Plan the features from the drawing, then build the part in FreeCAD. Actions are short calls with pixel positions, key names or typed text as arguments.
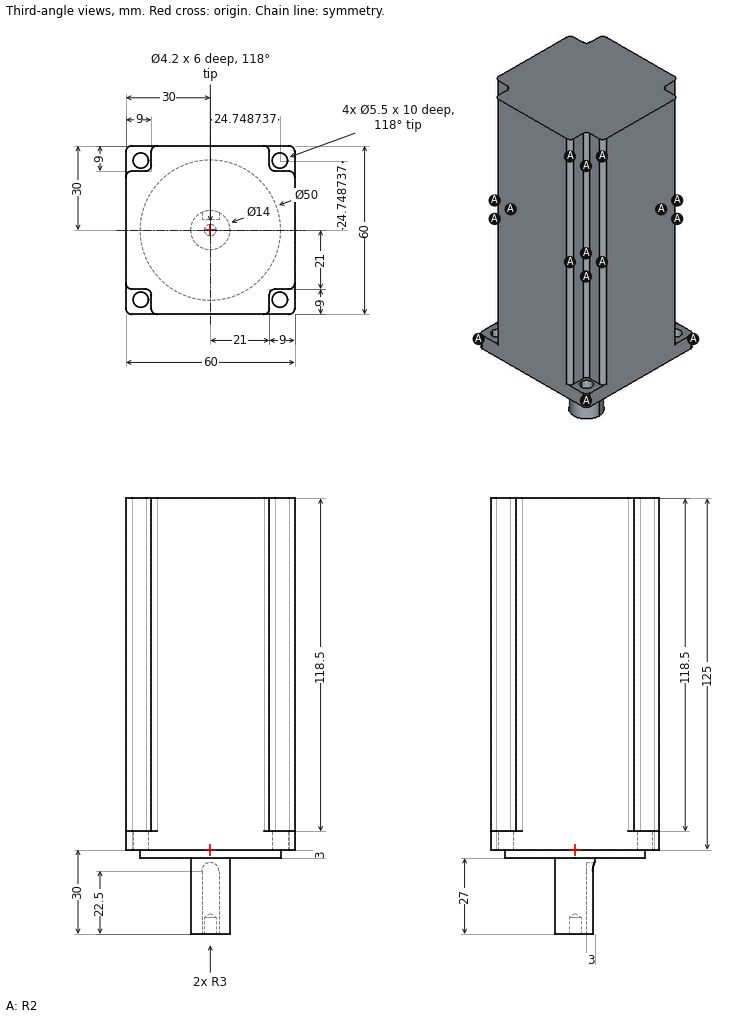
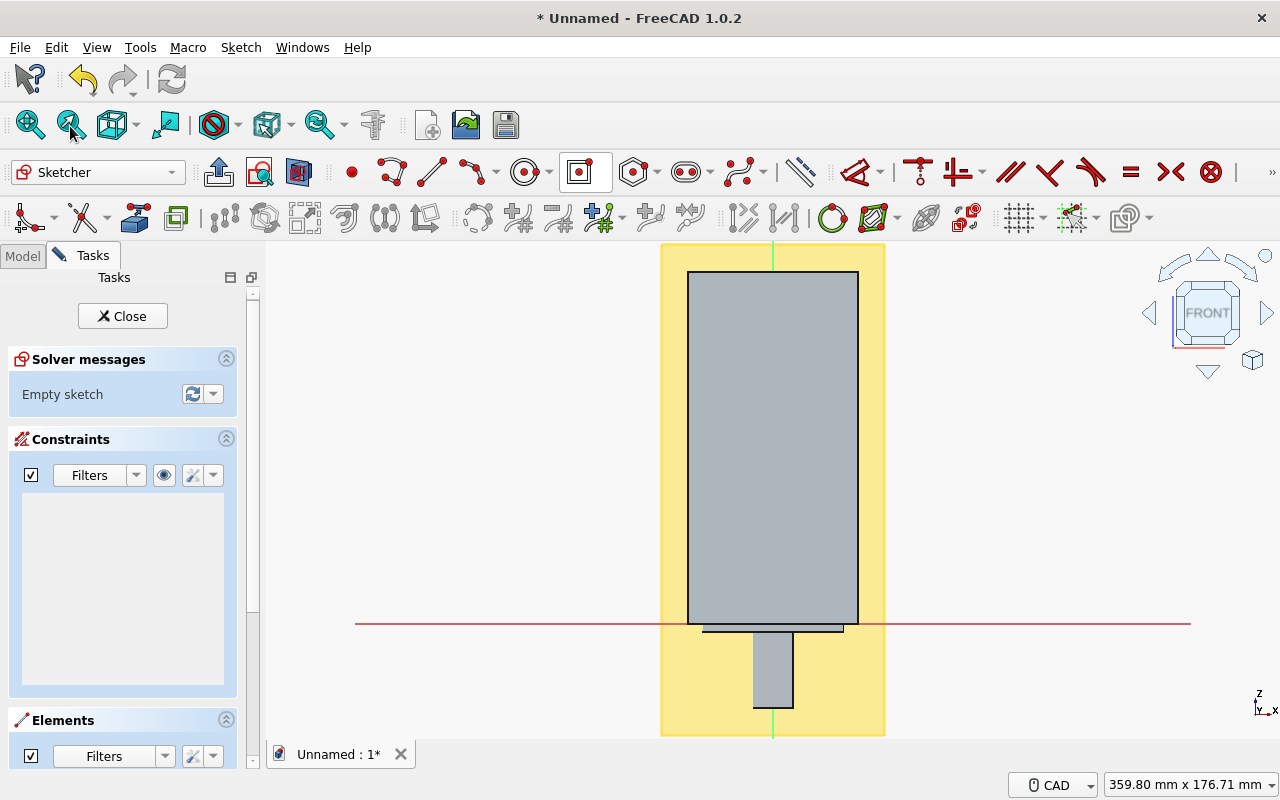
click(300, 172)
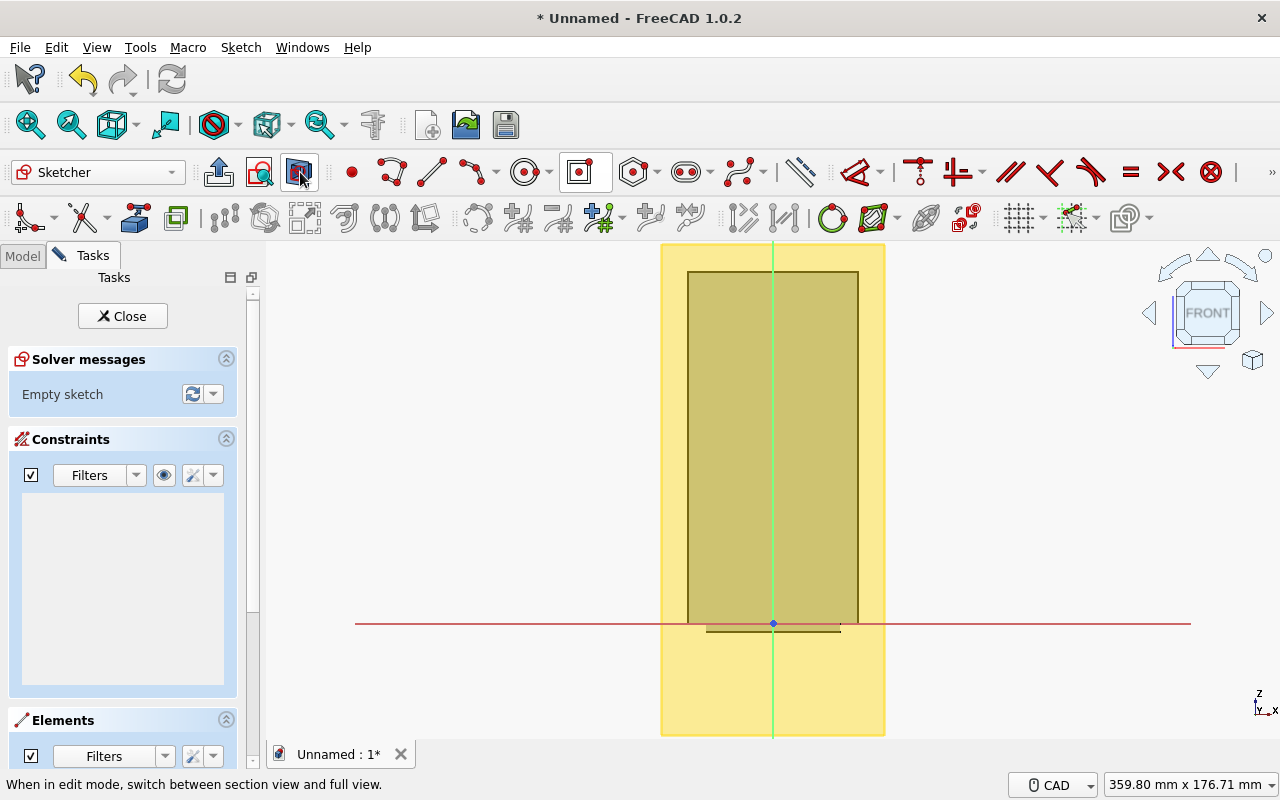
scroll(704, 490, down, 5)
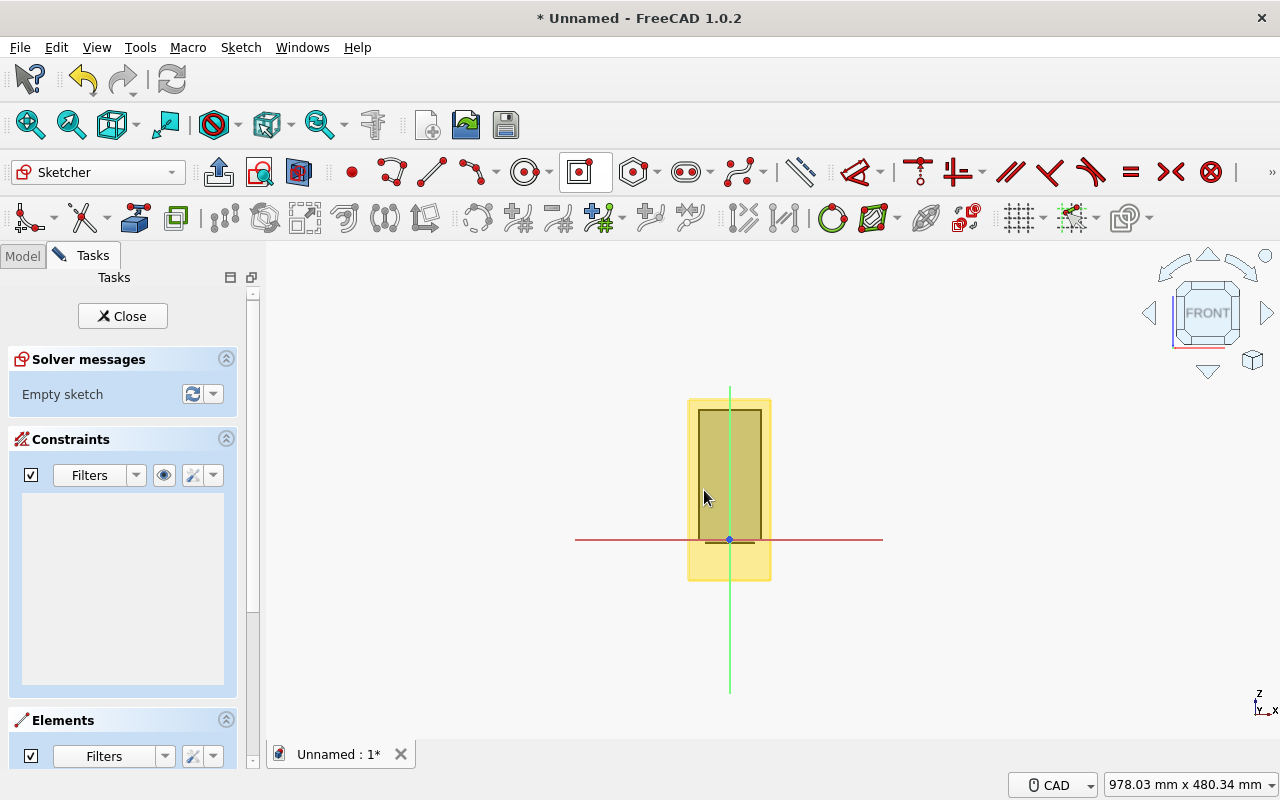
scroll(733, 565, up, 11)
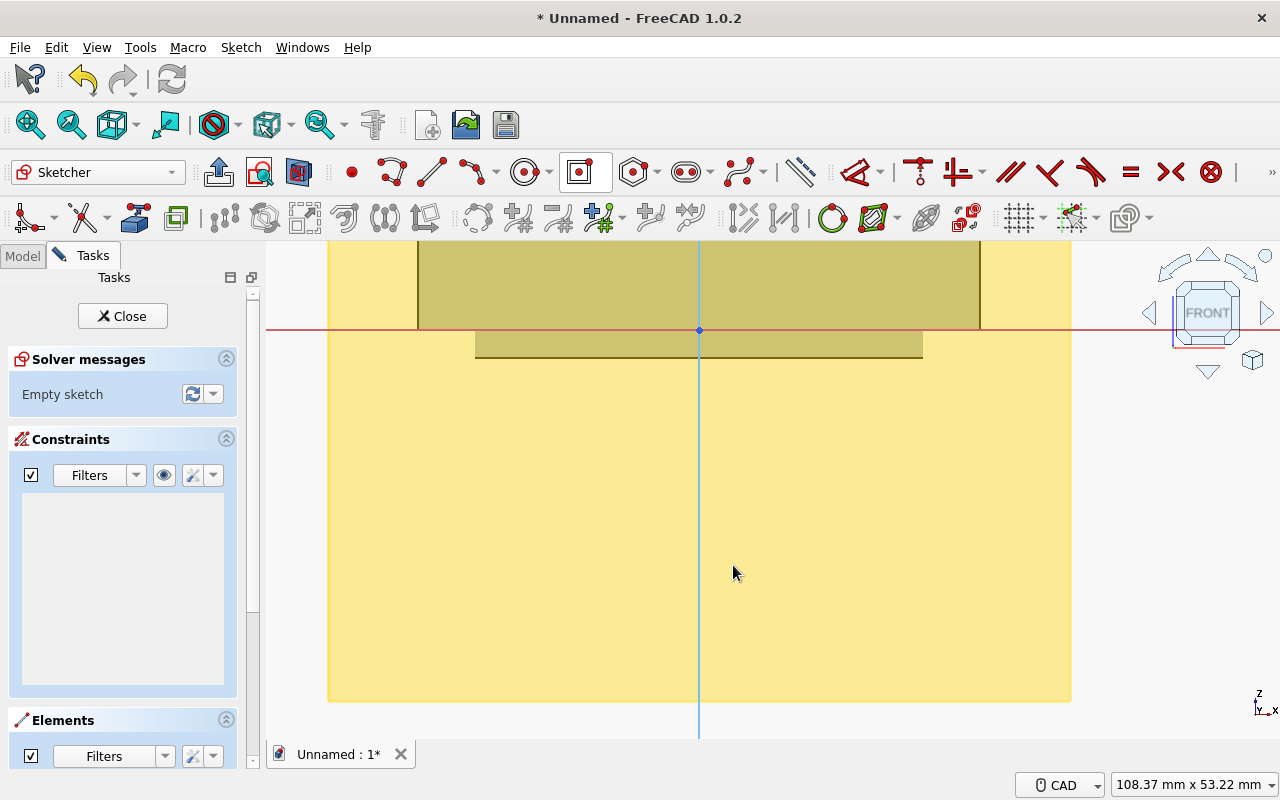
key(g)
key(s)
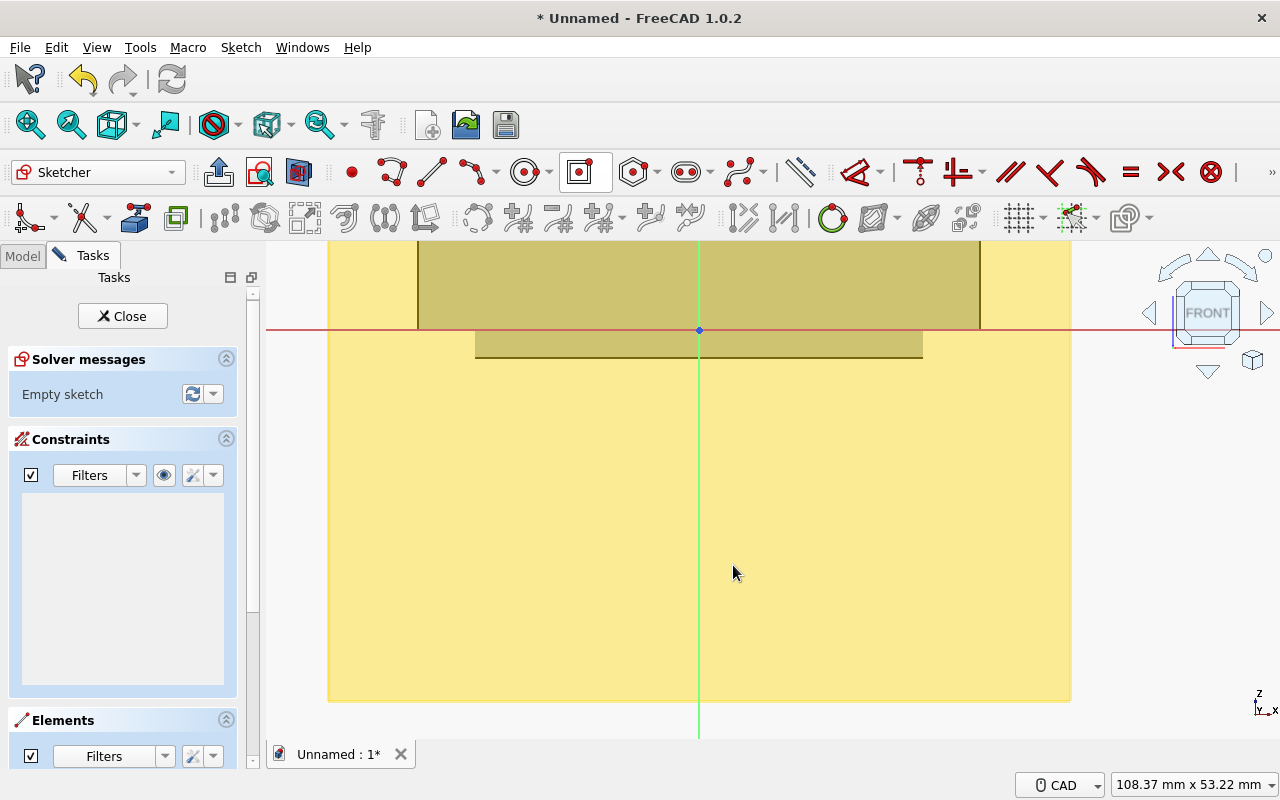
click(699, 611)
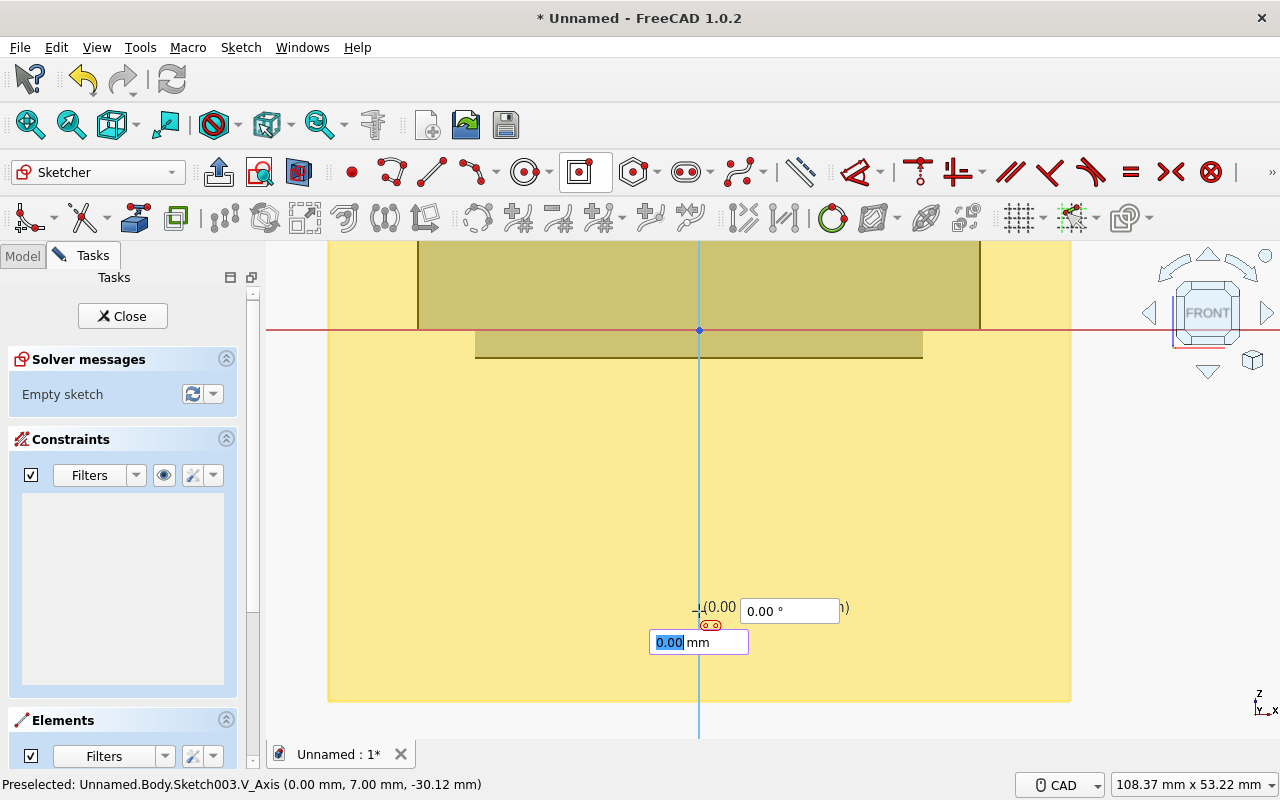
click(708, 400)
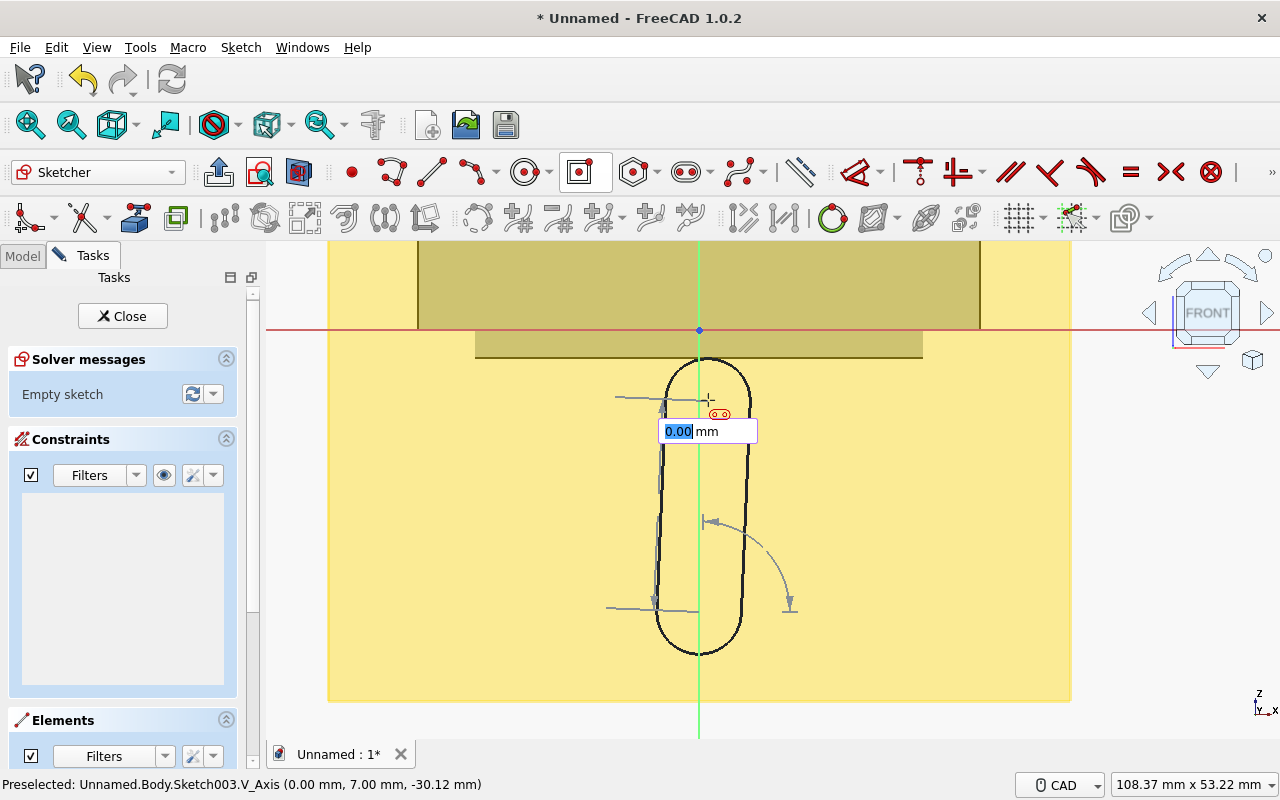
click(727, 506)
key(Escape)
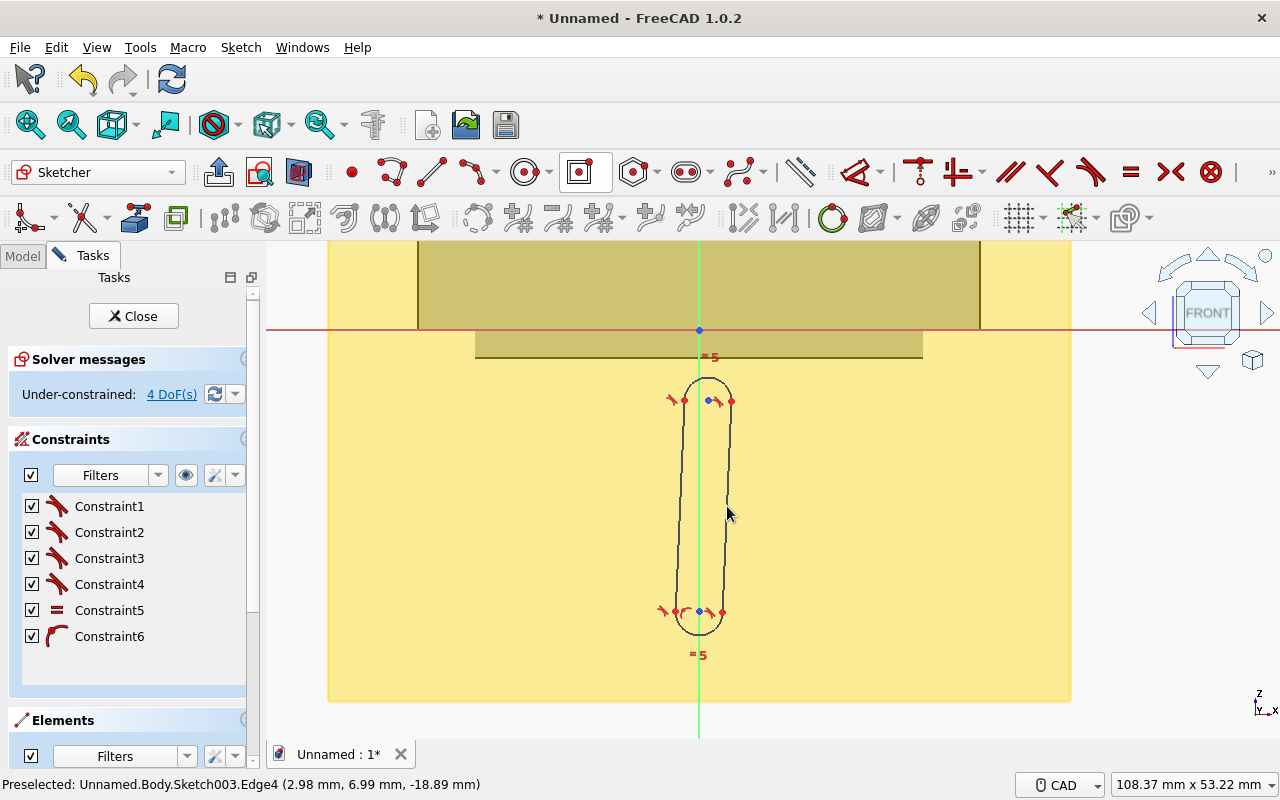
click(678, 548)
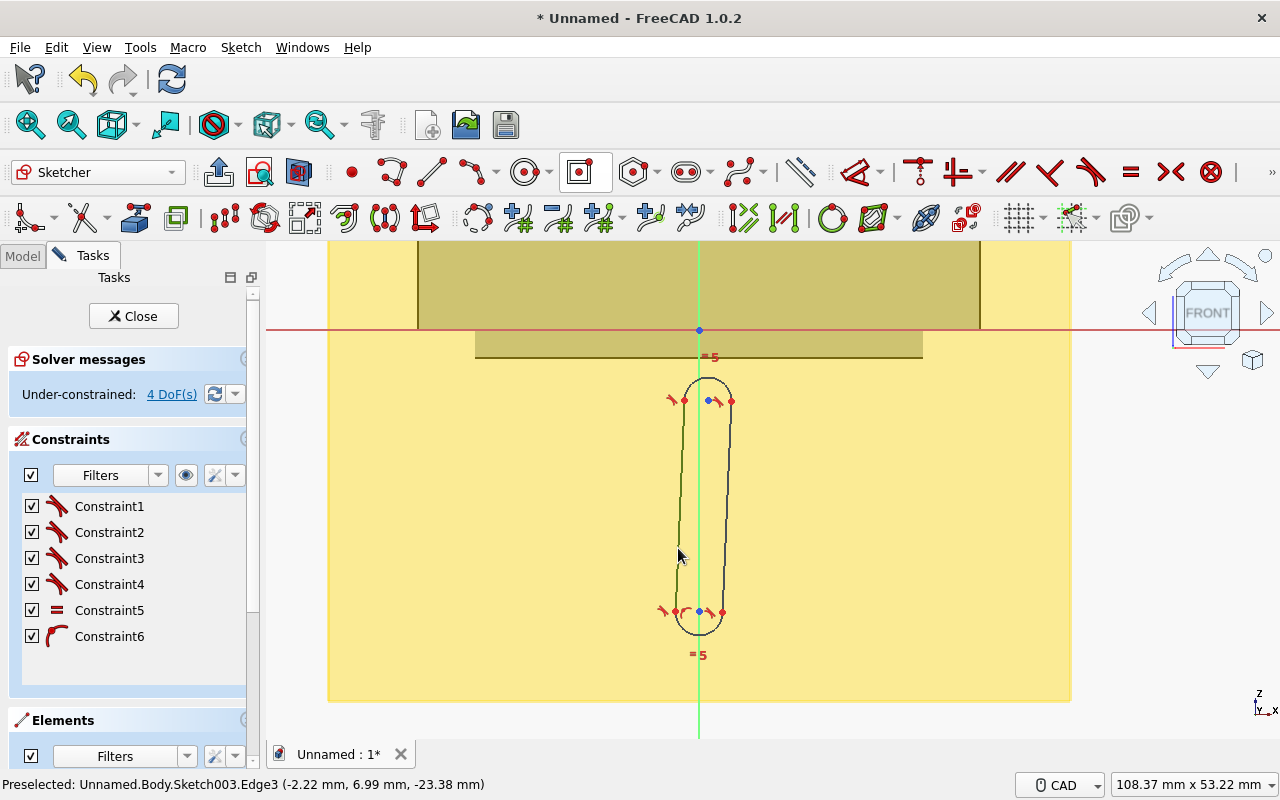
key(v)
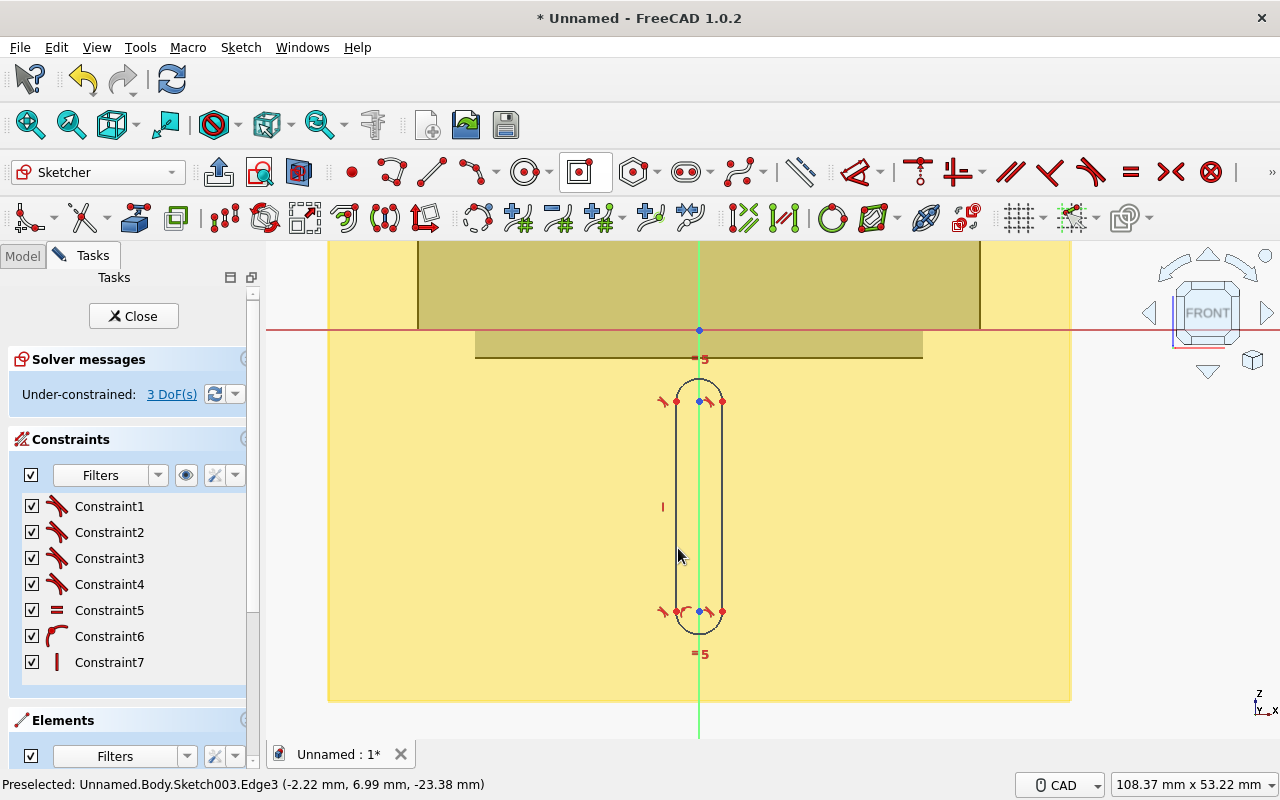
key(d)